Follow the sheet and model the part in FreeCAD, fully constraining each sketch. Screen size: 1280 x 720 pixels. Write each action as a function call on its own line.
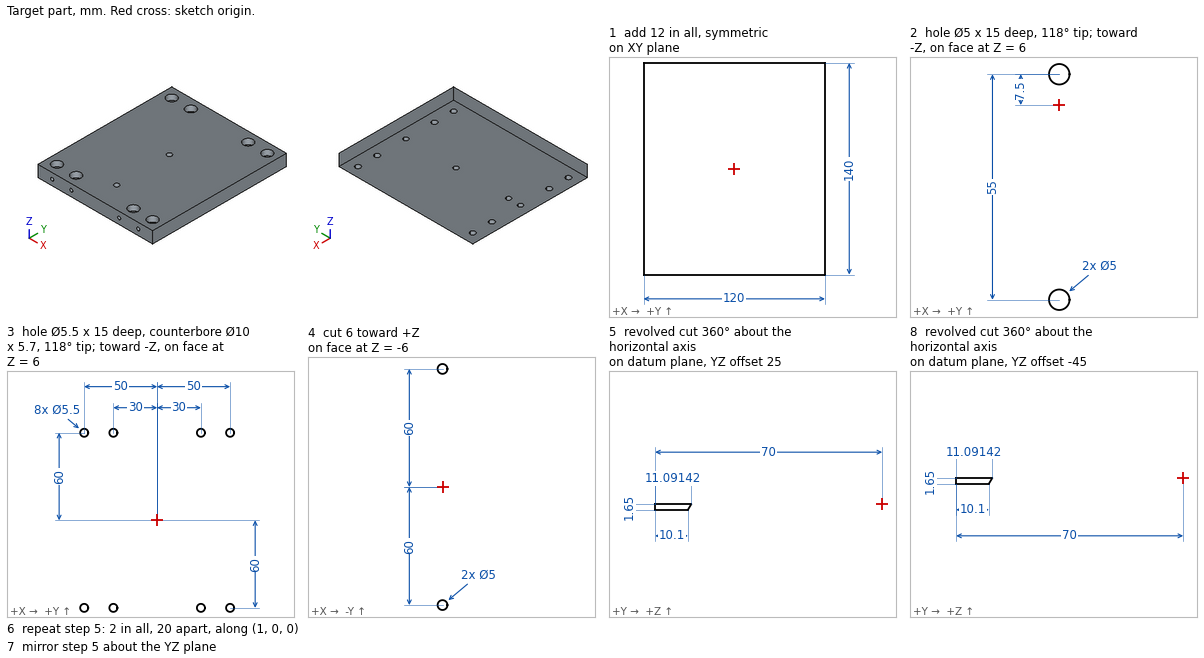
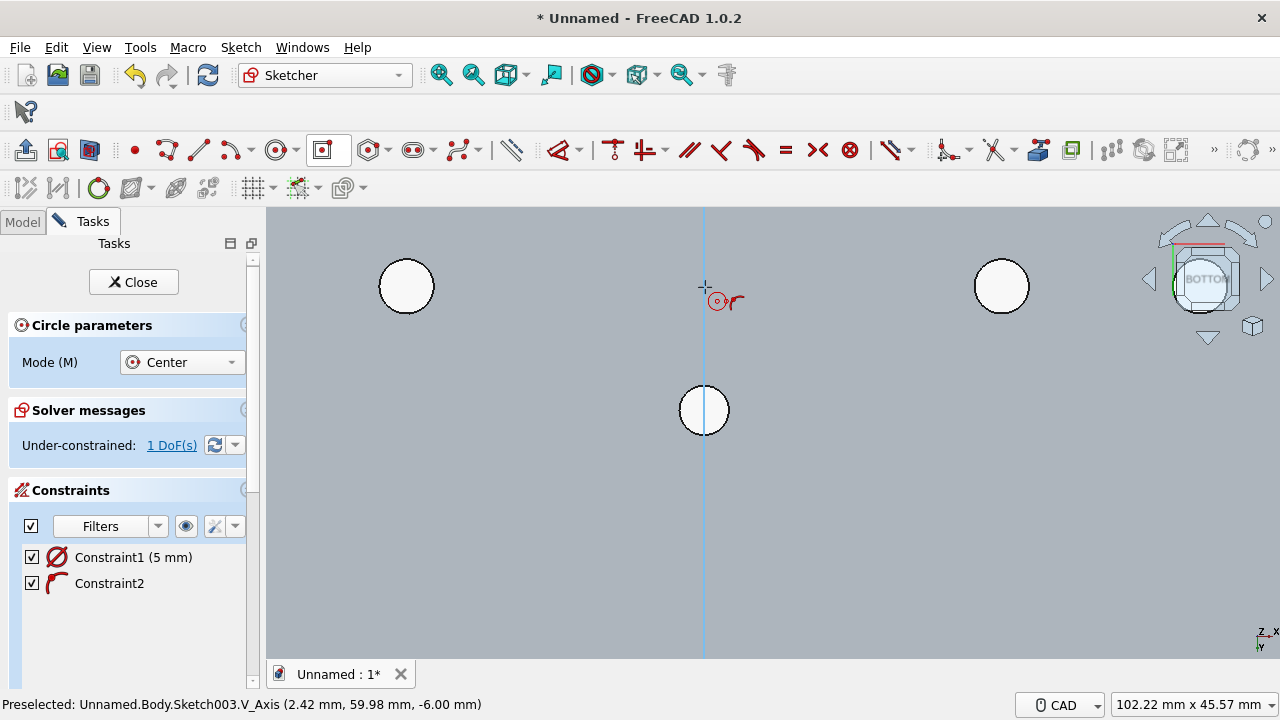
scroll(705, 286, down, 7)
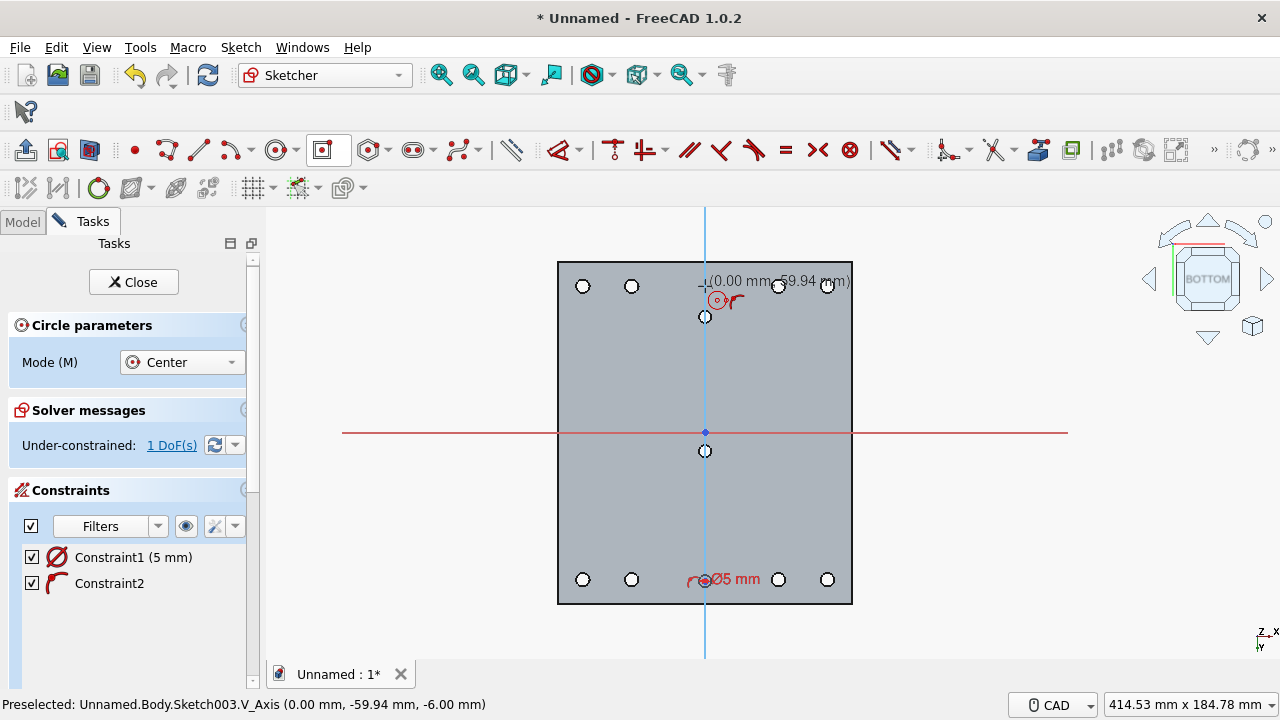
click(705, 286)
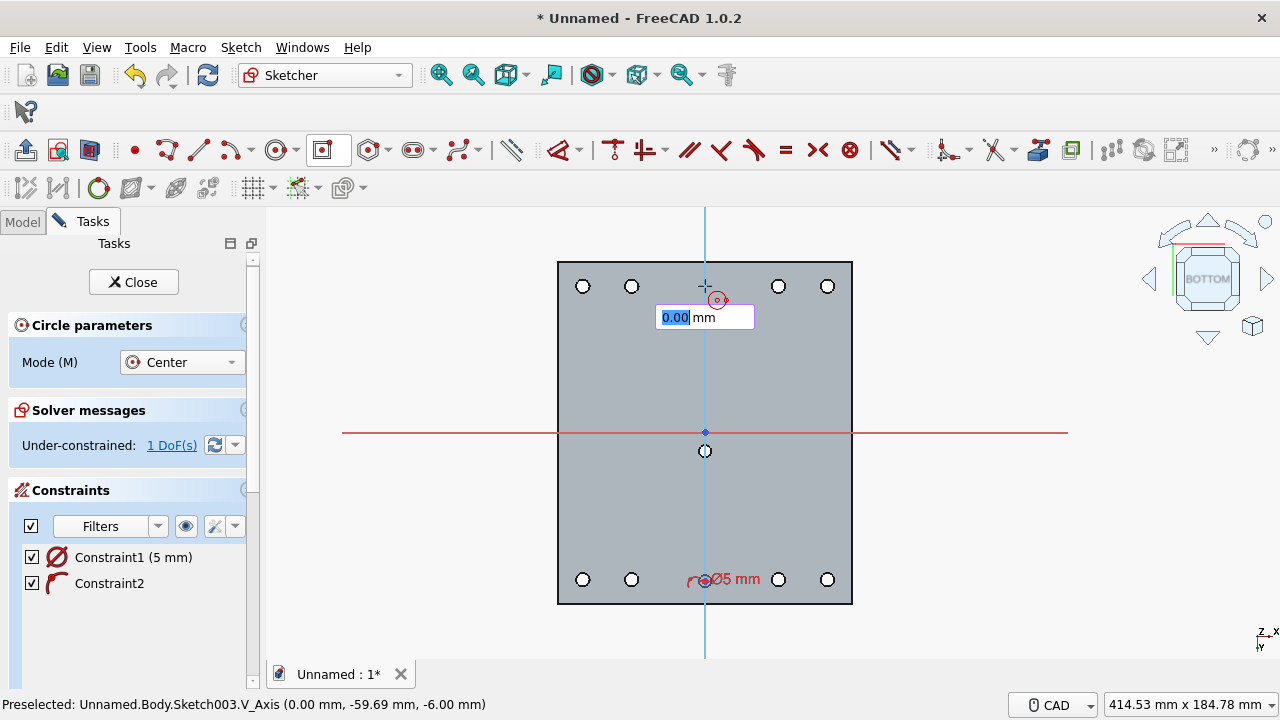
scroll(711, 284, up, 6)
move(710, 284)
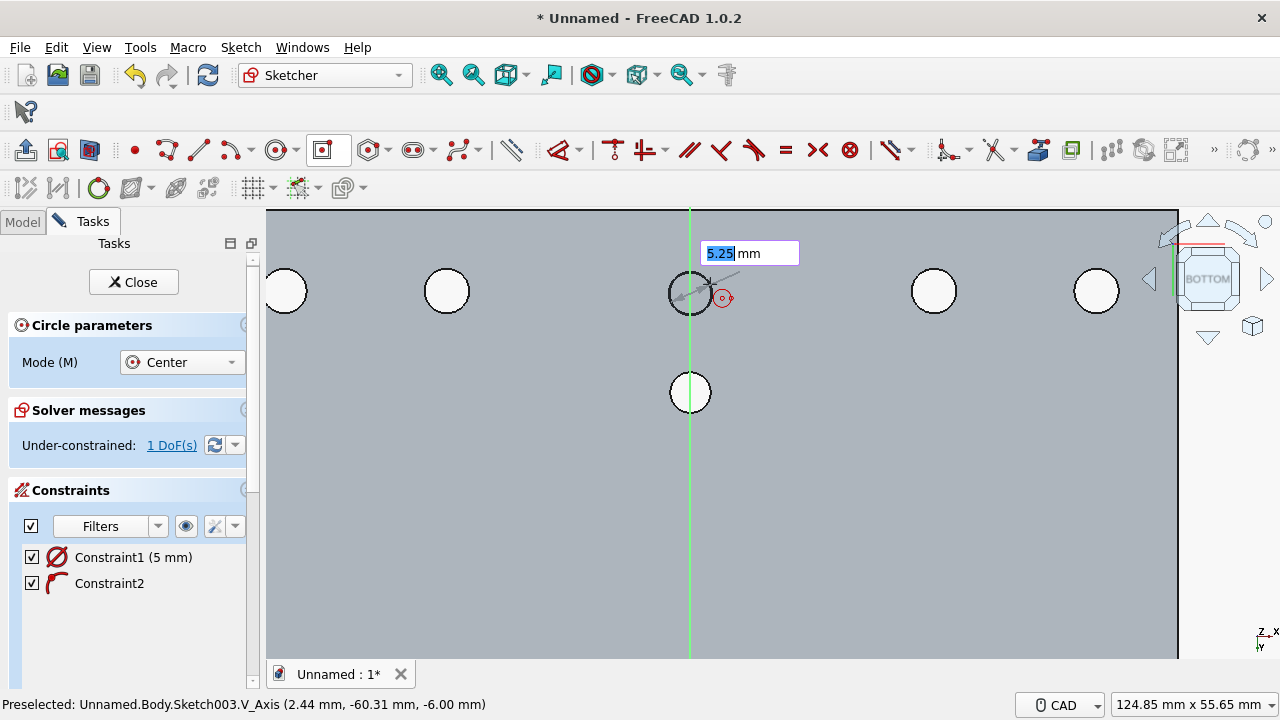
text(5)
key(Return)
key(Escape)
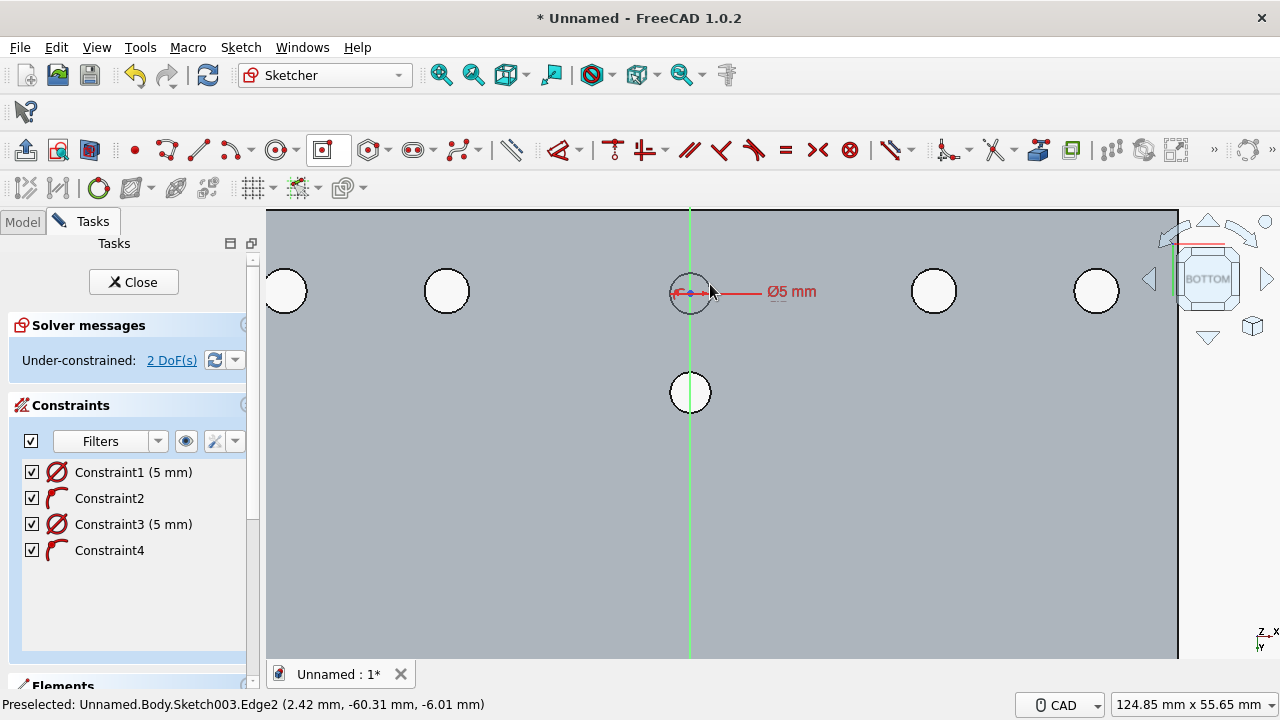
key(d)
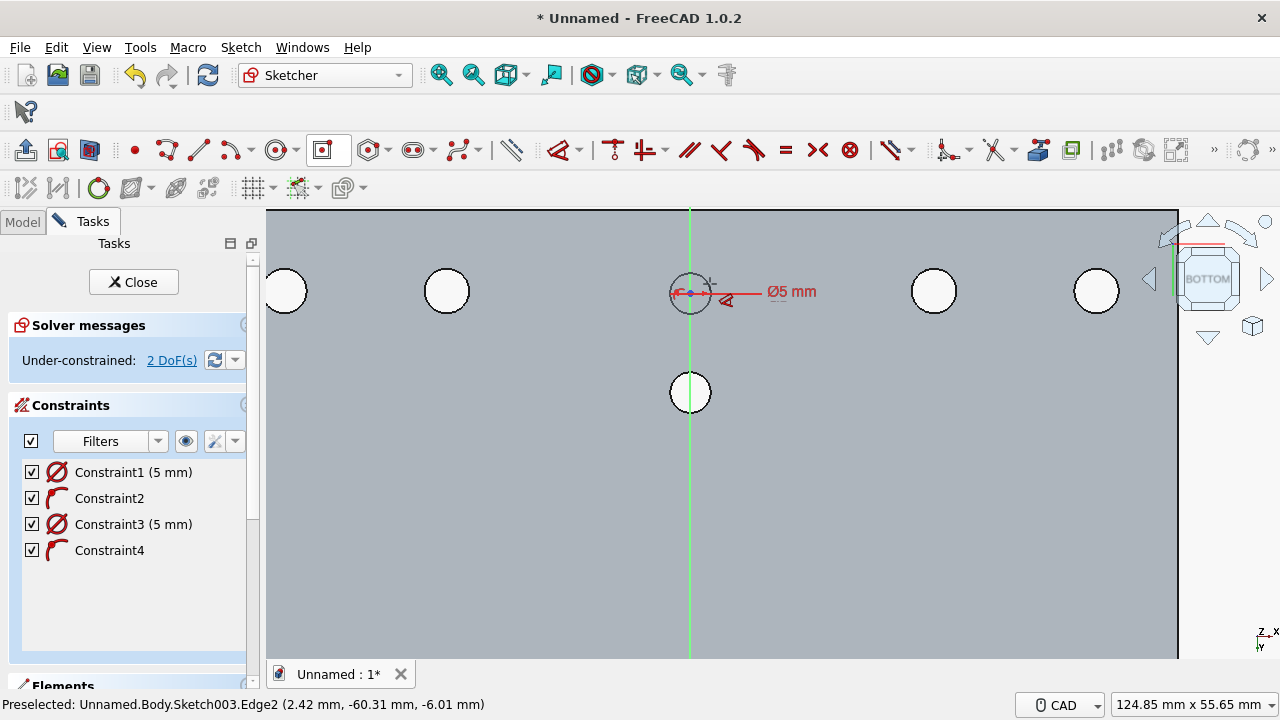
scroll(711, 284, down, 6)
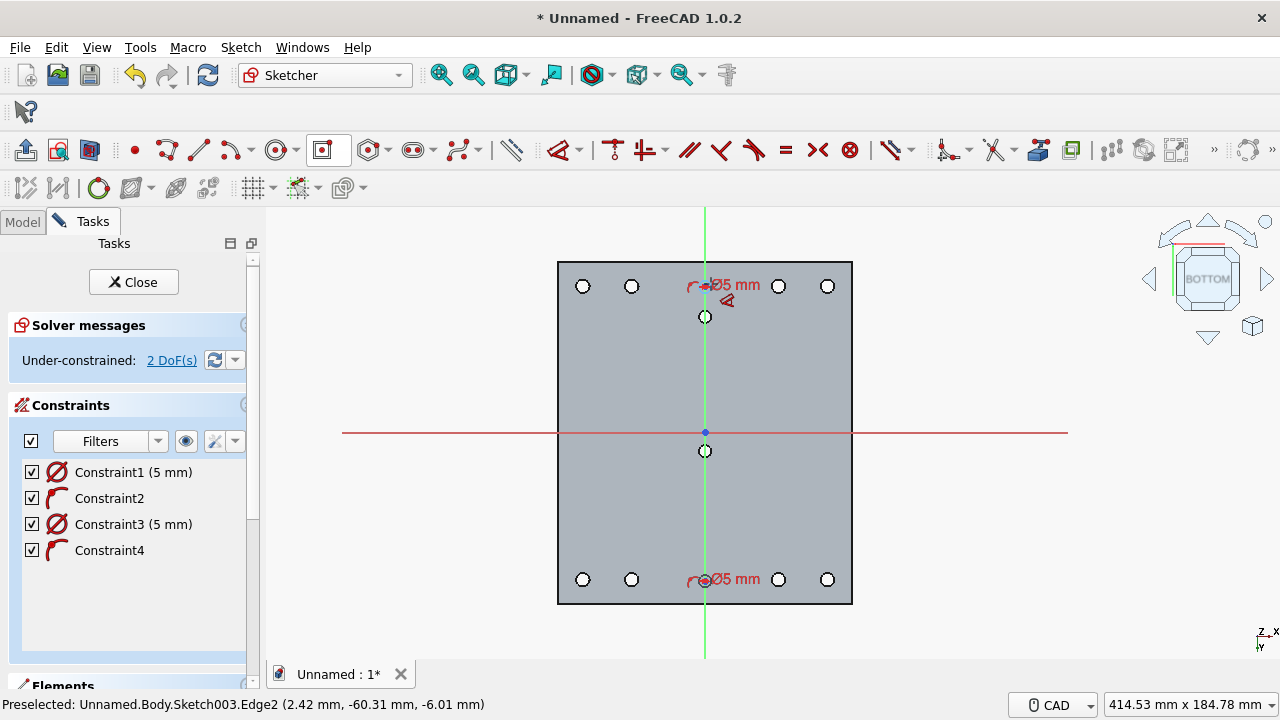
click(705, 581)
click(739, 507)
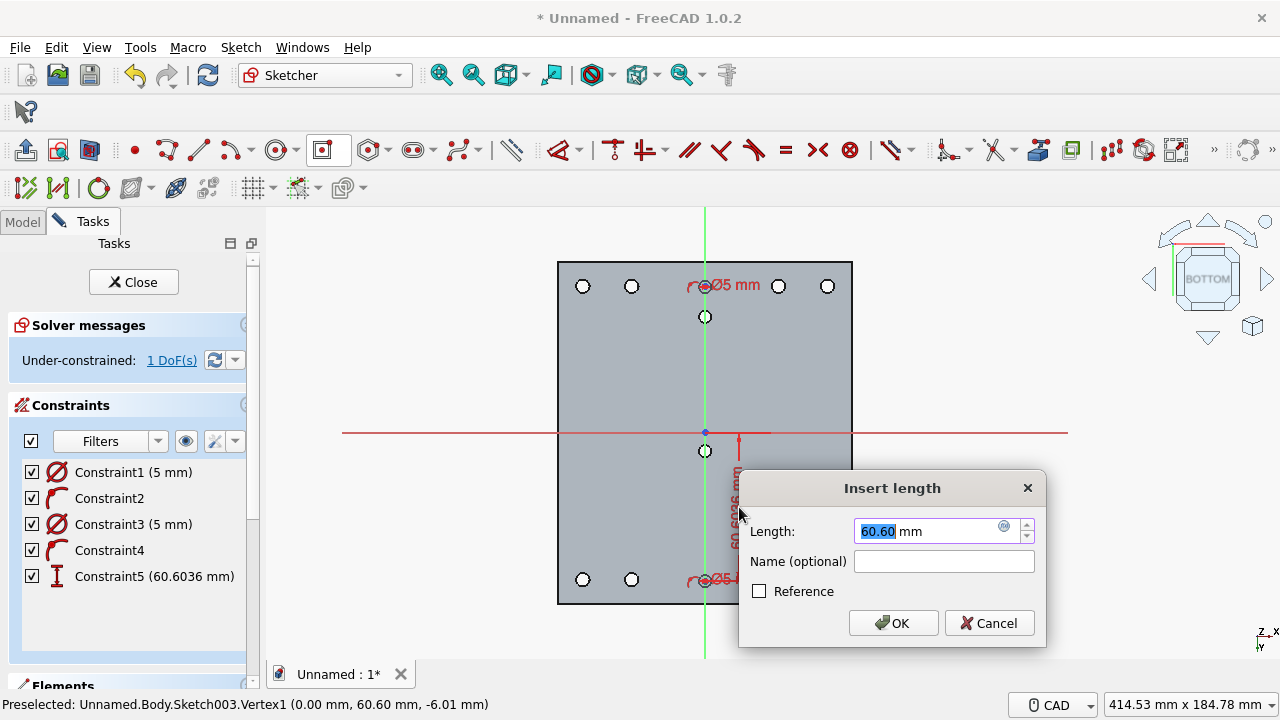
text(60)
key(Return)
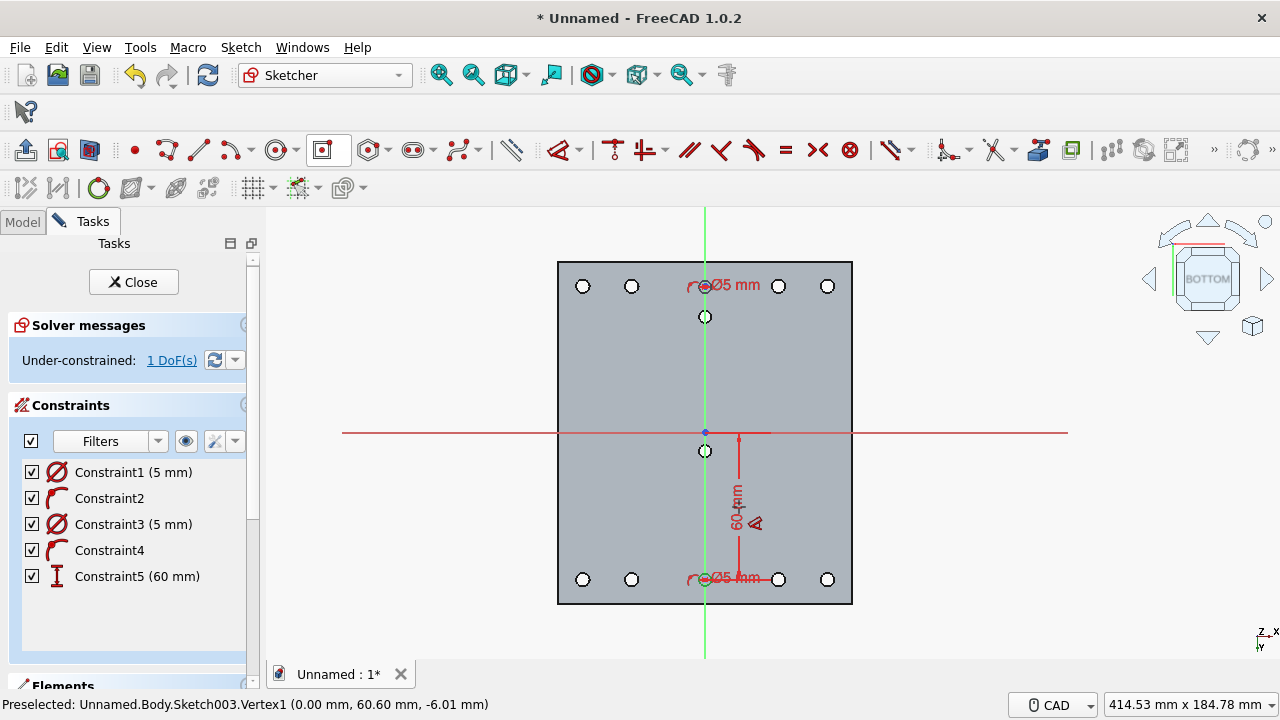
click(705, 287)
click(739, 360)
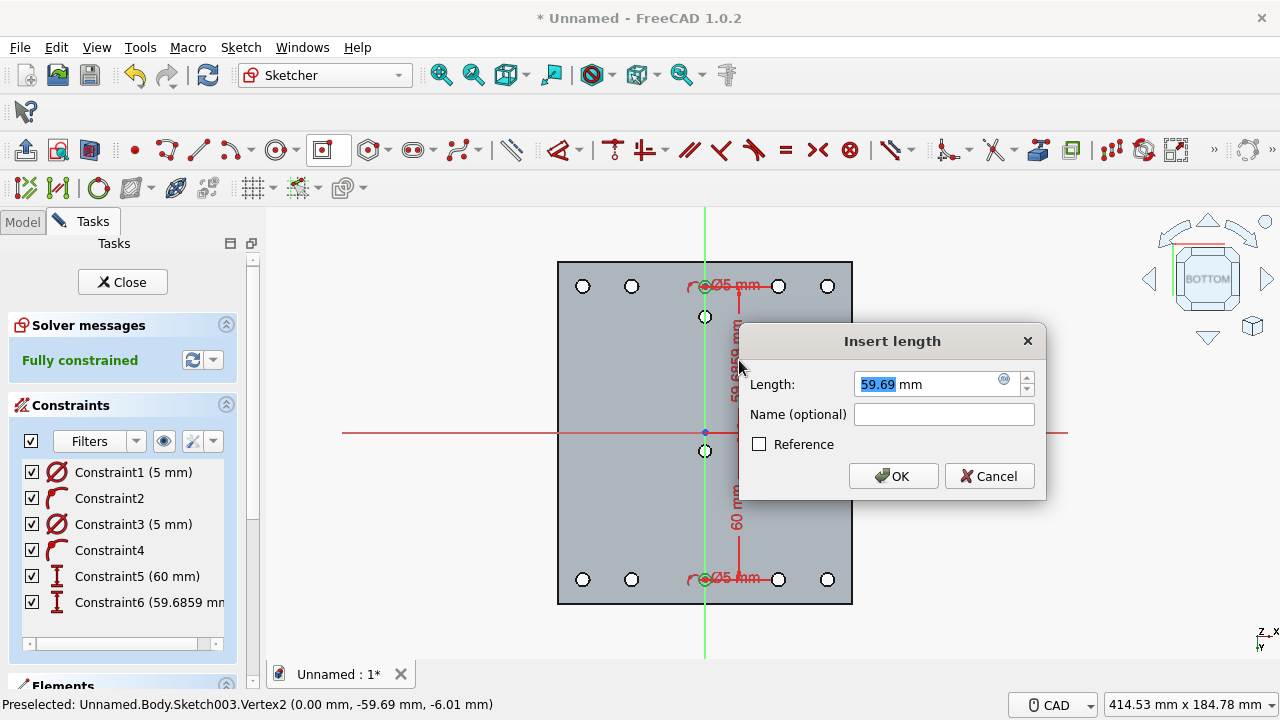
text(60)
key(Return)
key(Escape)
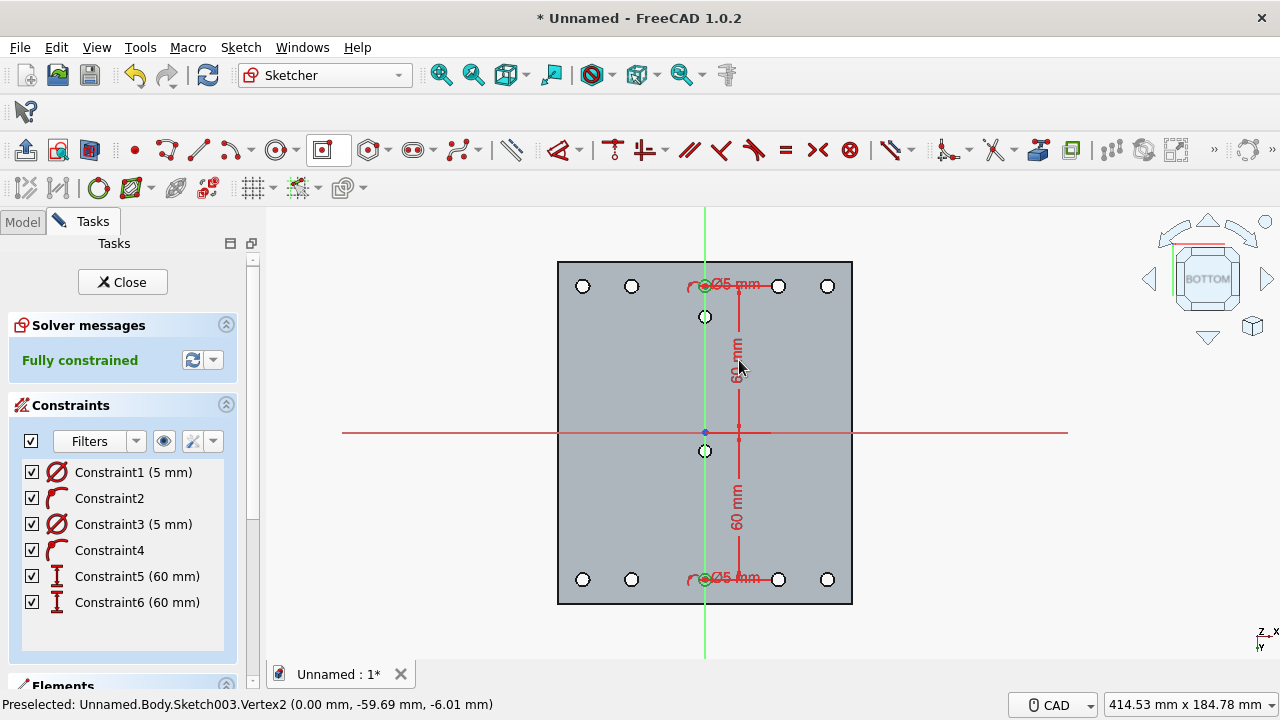
click(123, 282)